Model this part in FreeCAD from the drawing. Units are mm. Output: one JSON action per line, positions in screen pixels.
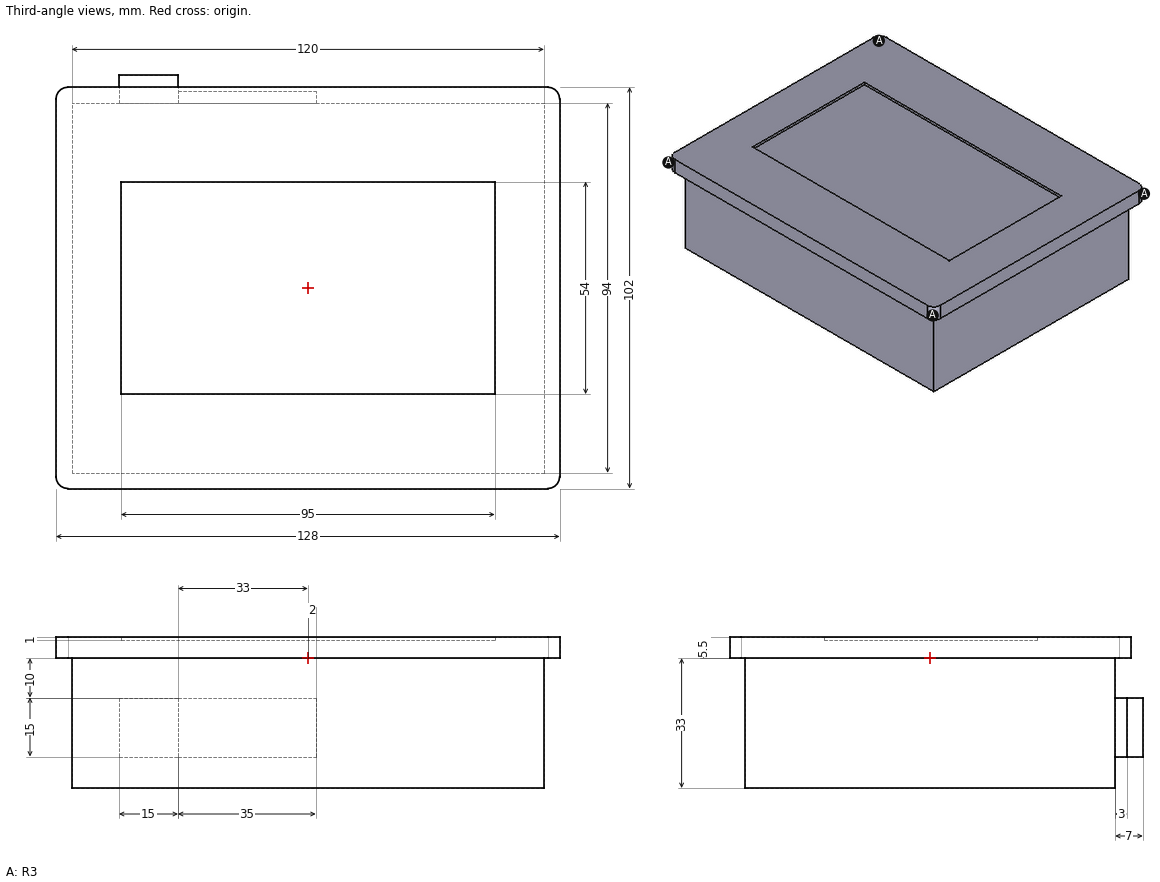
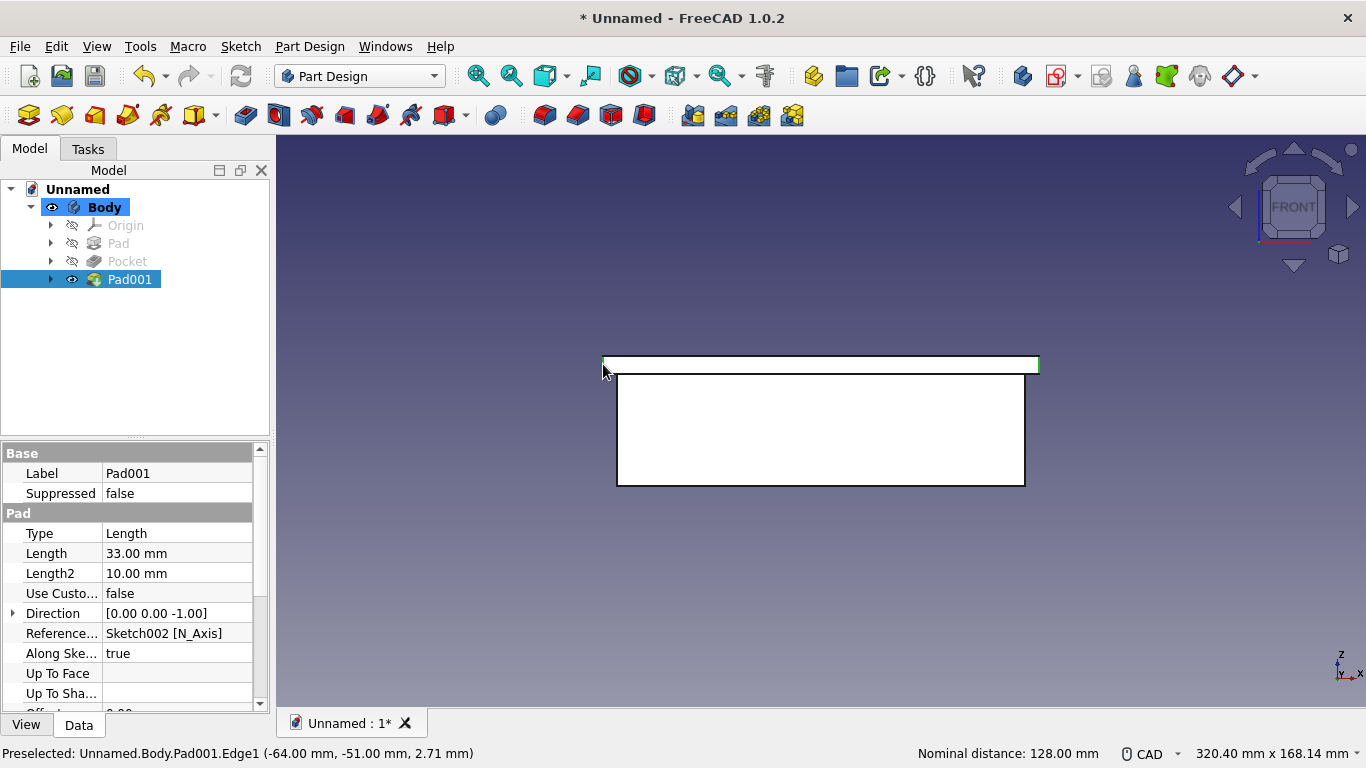
{"action": "scroll", "coordinate": [603, 364], "scroll_direction": "up", "scroll_amount": 4}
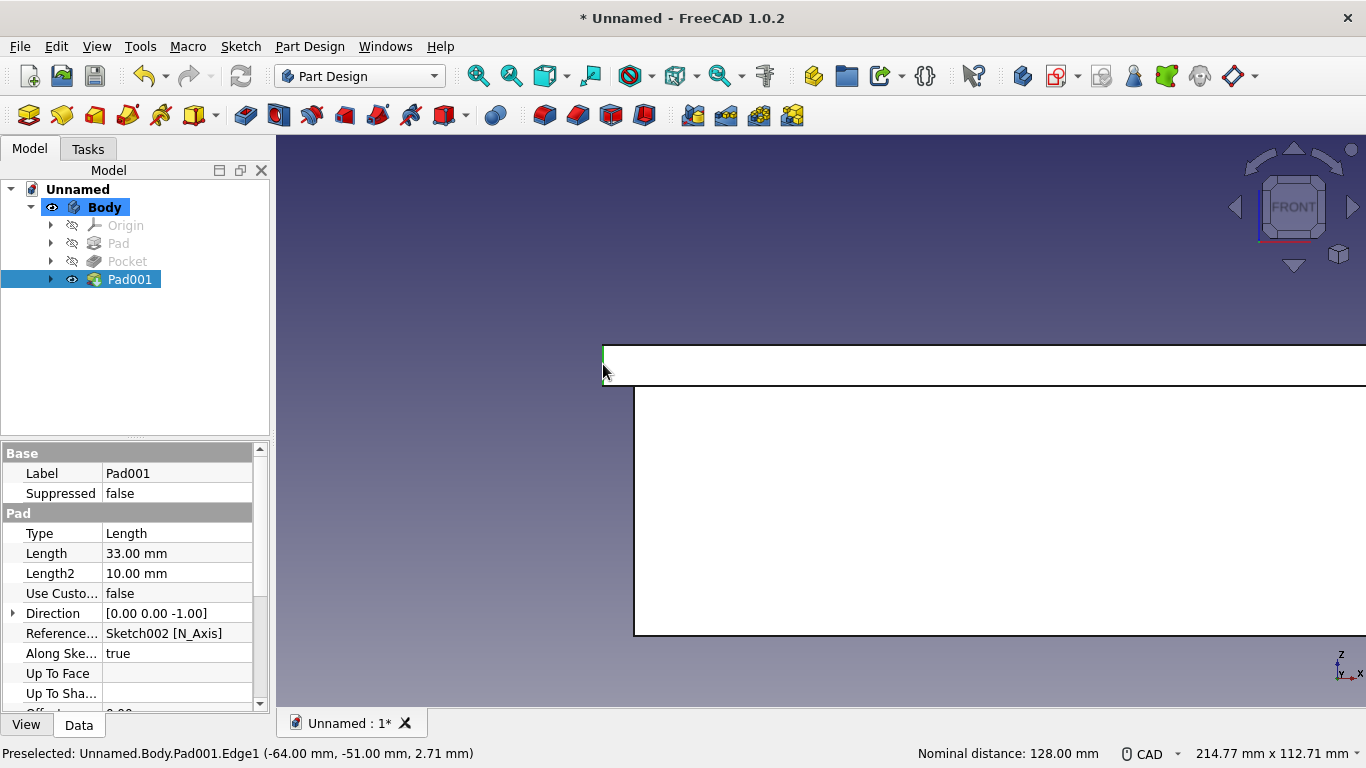
{"action": "left_click", "coordinate": [479, 76]}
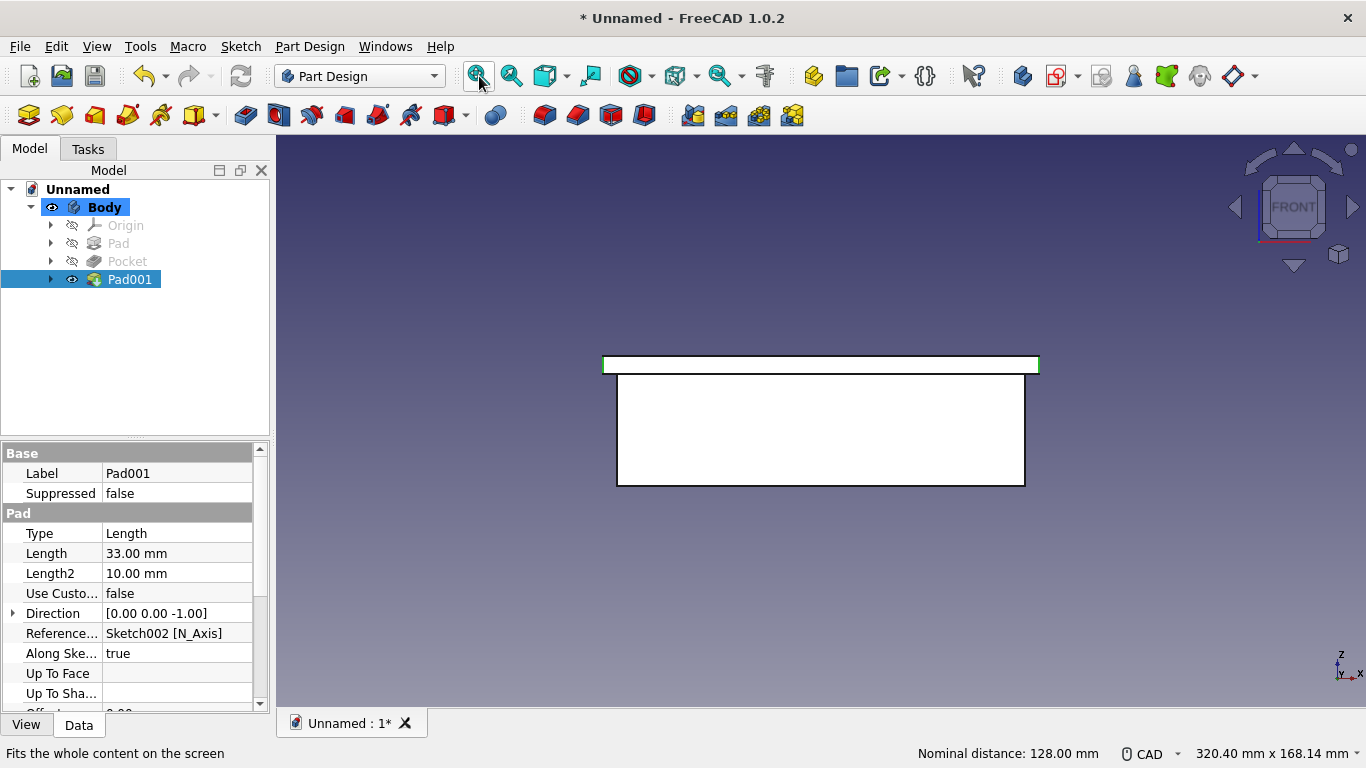
{"action": "key", "text": "3"}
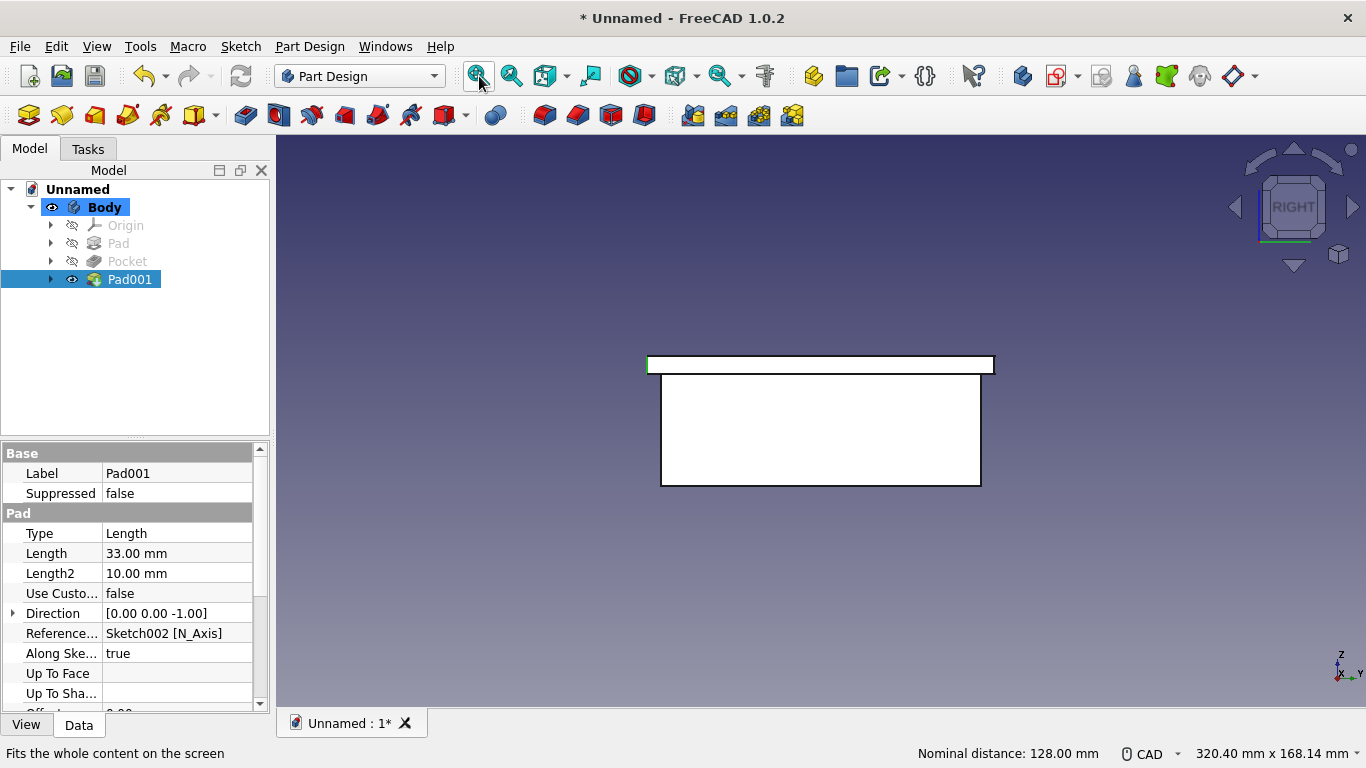
{"action": "key", "text": "v f"}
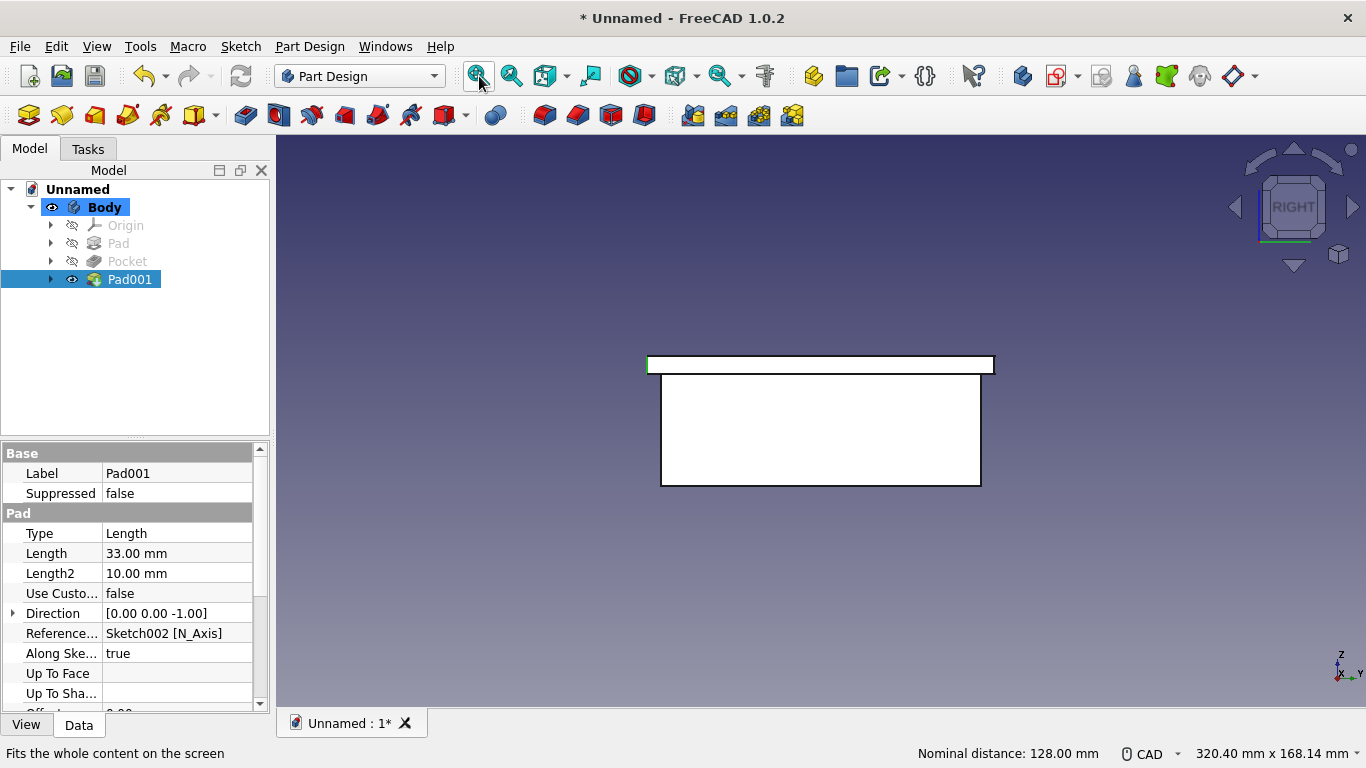
{"action": "left_click", "coordinate": [995, 364], "text": "ctrl"}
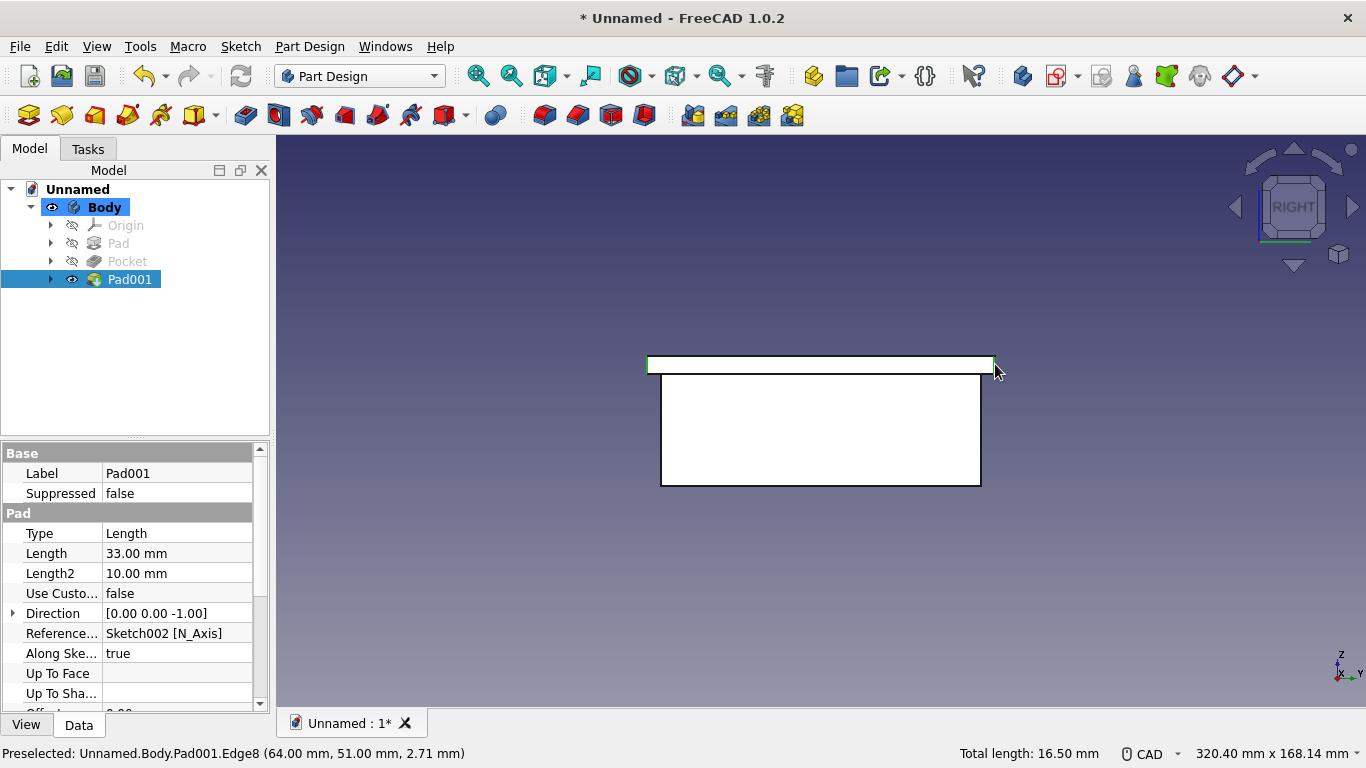
{"action": "scroll", "coordinate": [995, 364], "scroll_direction": "up", "scroll_amount": 4}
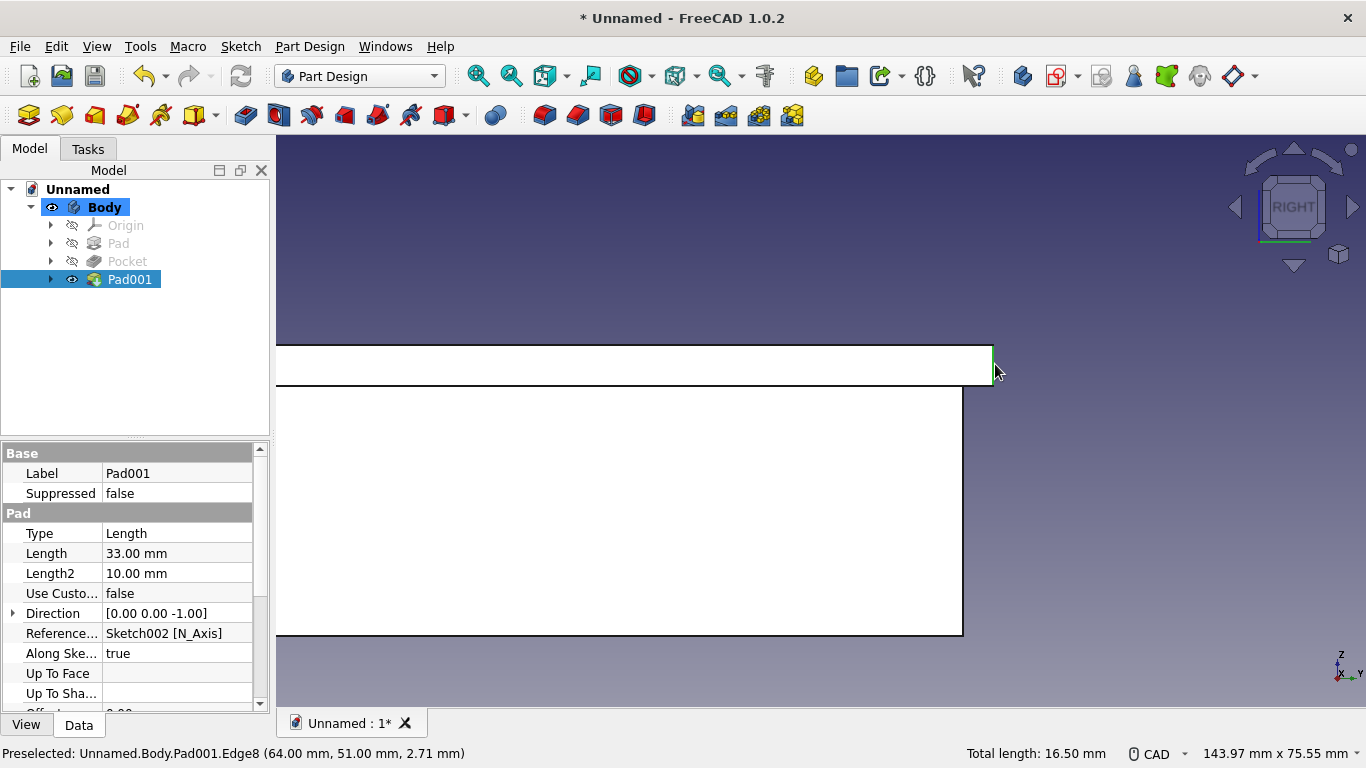
{"action": "key", "text": "v f"}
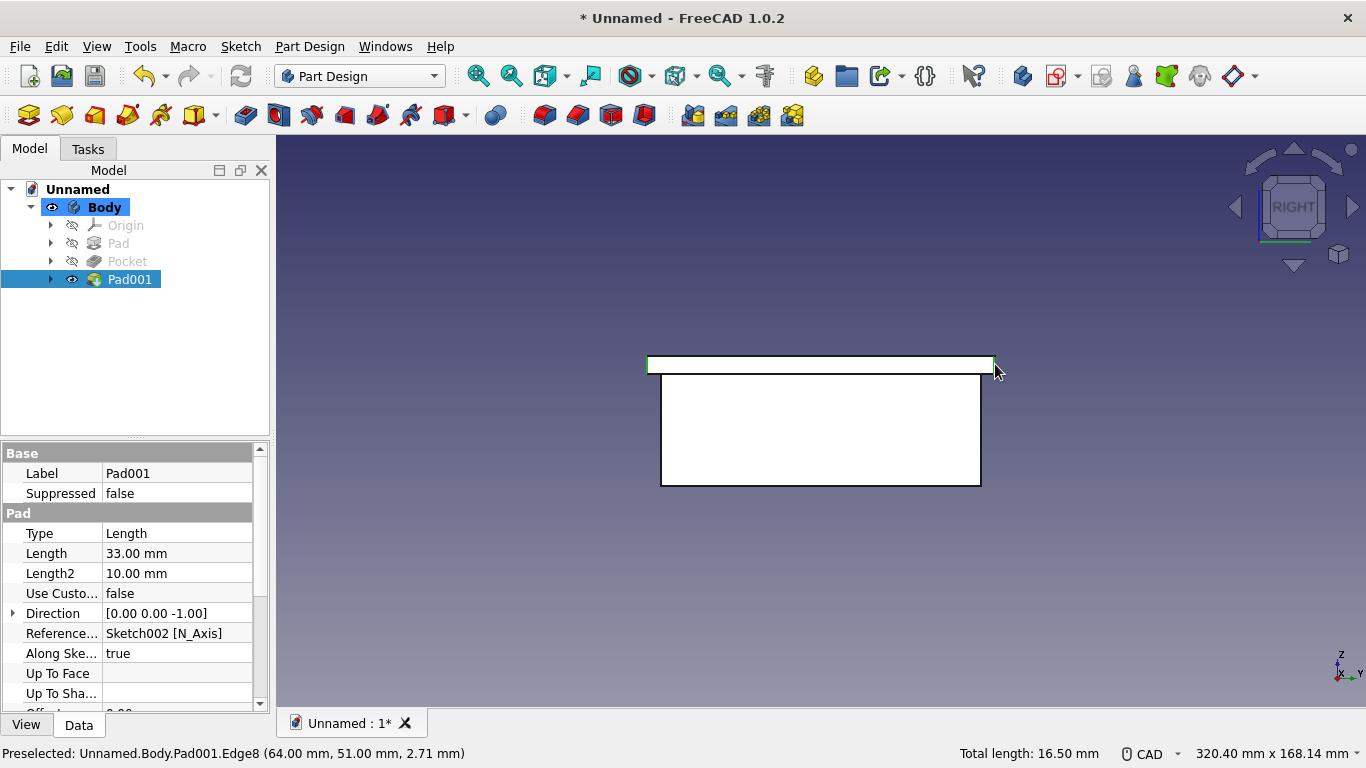
{"action": "key", "text": "5"}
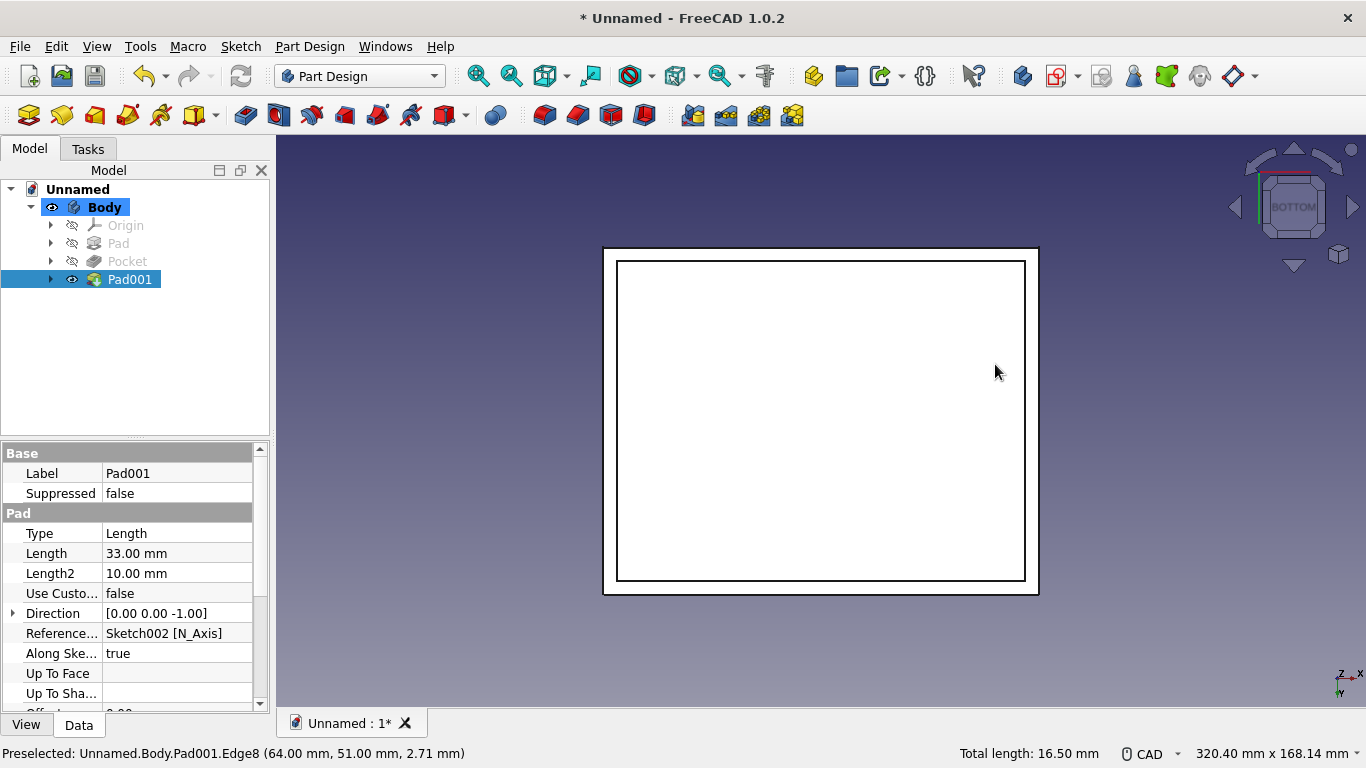
{"action": "scroll", "coordinate": [603, 594], "scroll_direction": "up", "scroll_amount": 4}